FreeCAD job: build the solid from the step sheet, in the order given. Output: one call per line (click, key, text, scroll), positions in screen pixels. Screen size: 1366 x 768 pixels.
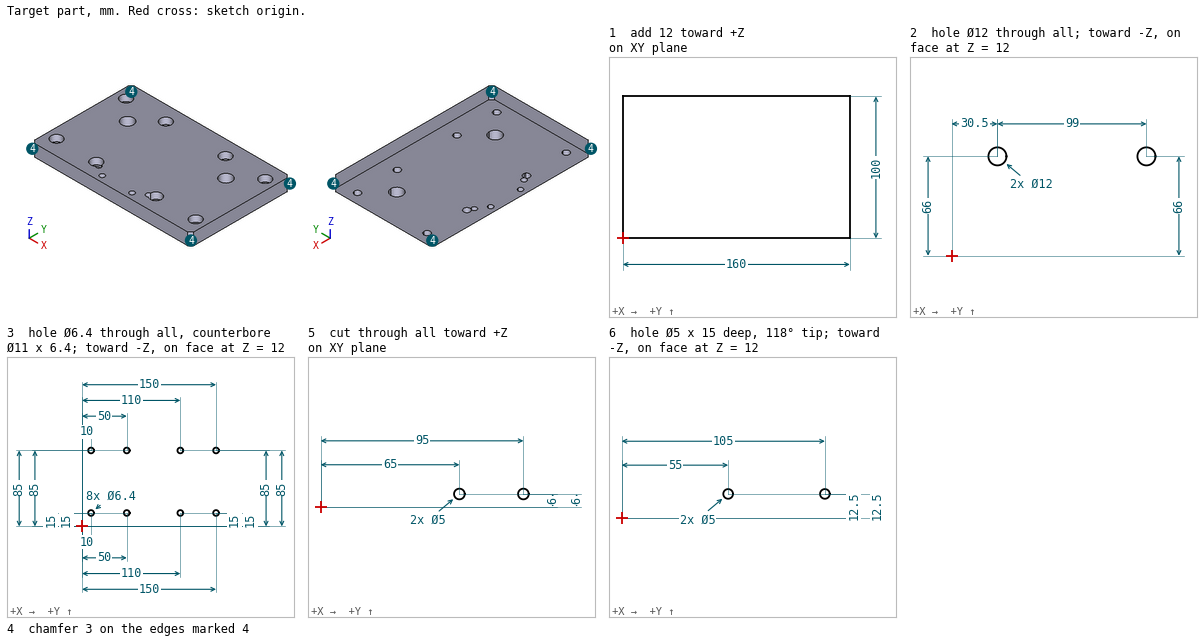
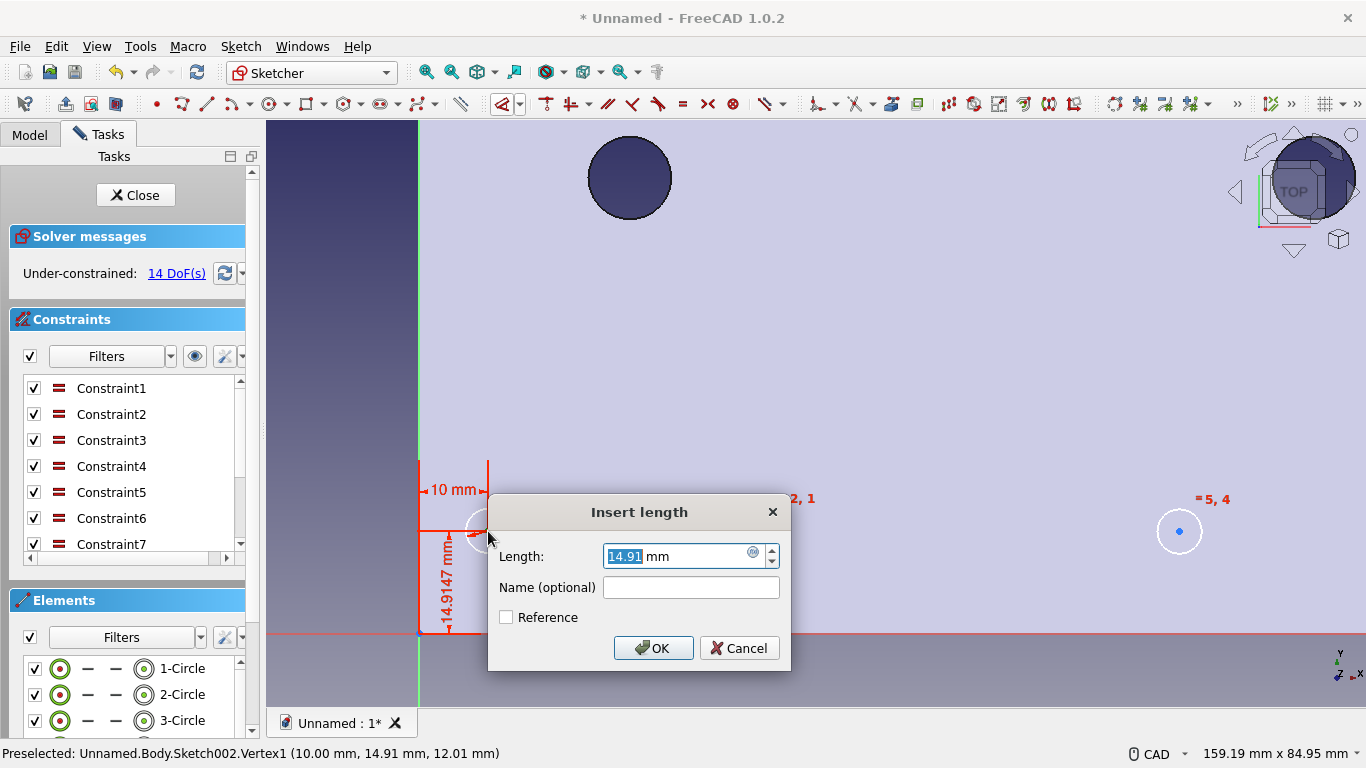
text(15)
key(Return)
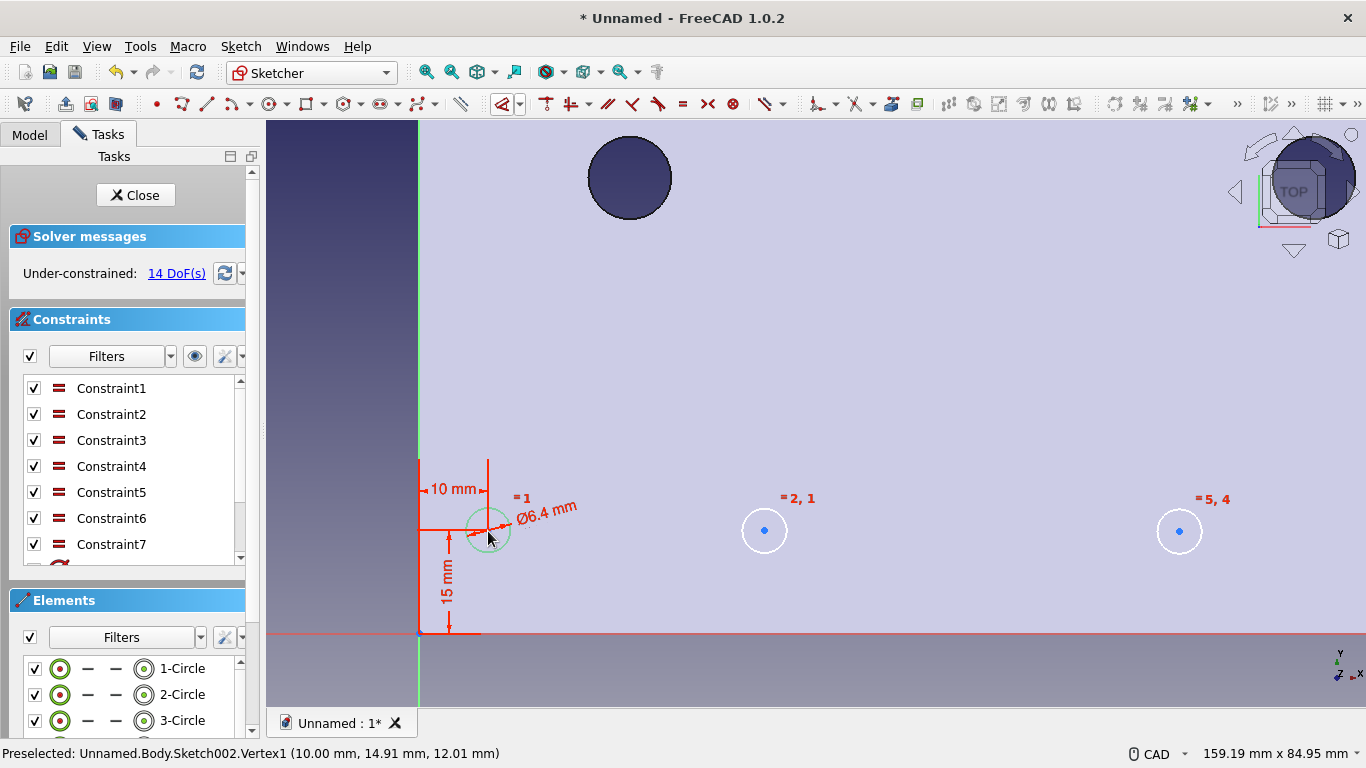
click(765, 531)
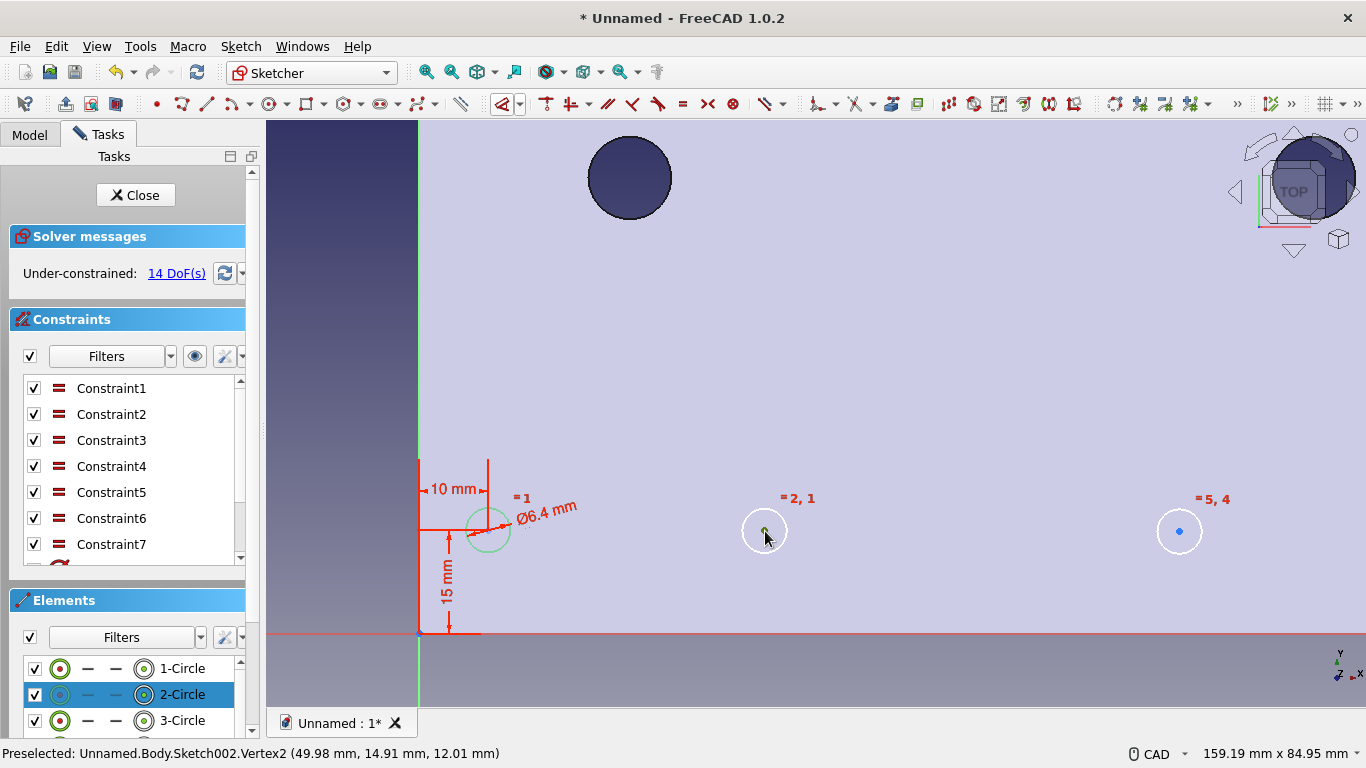
key(l)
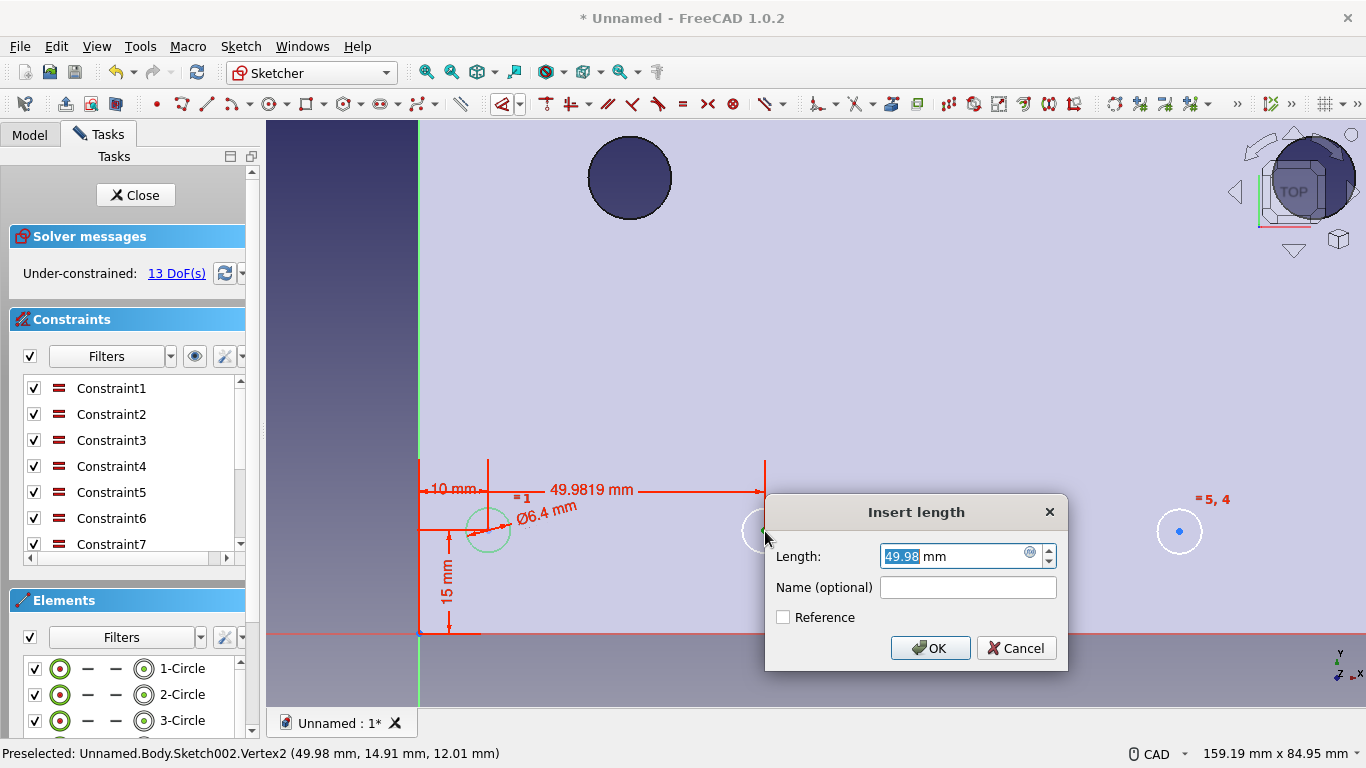
text(50)
key(Return)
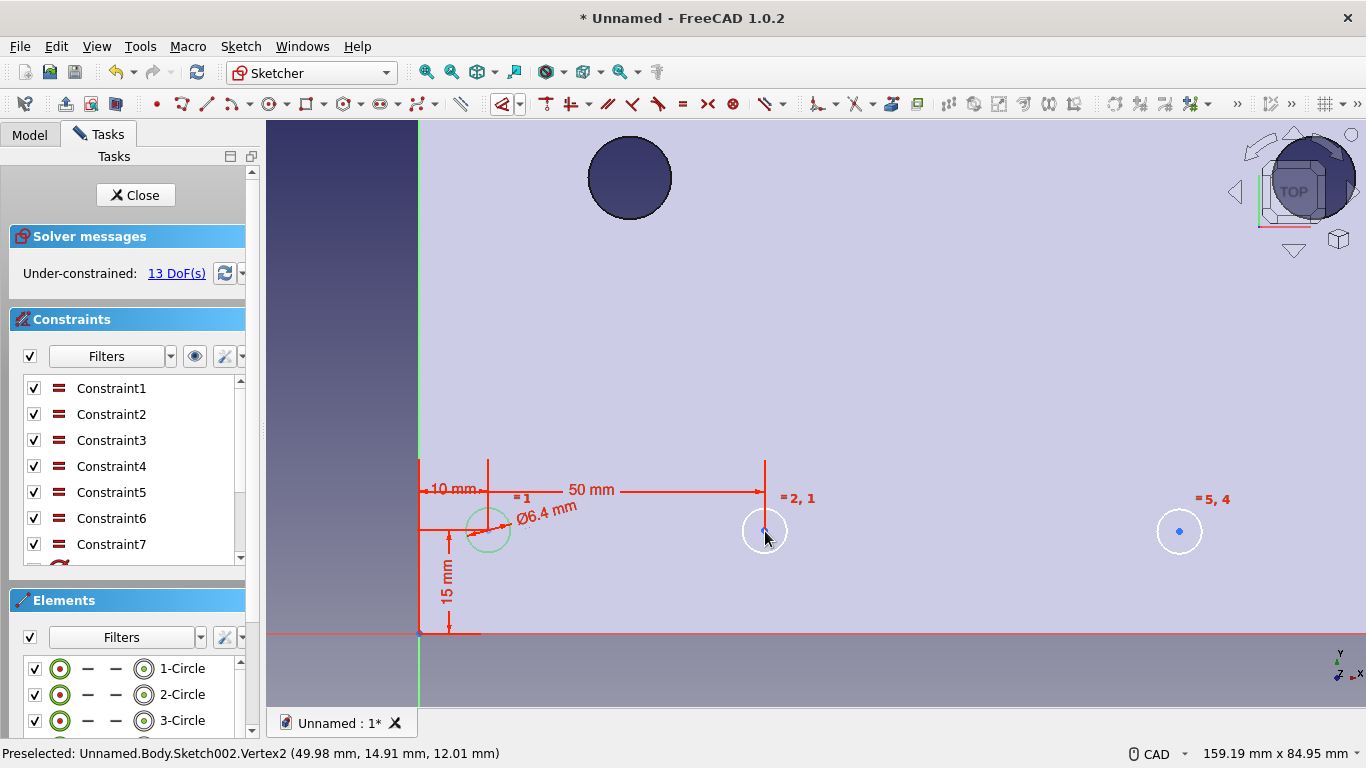
click(765, 531)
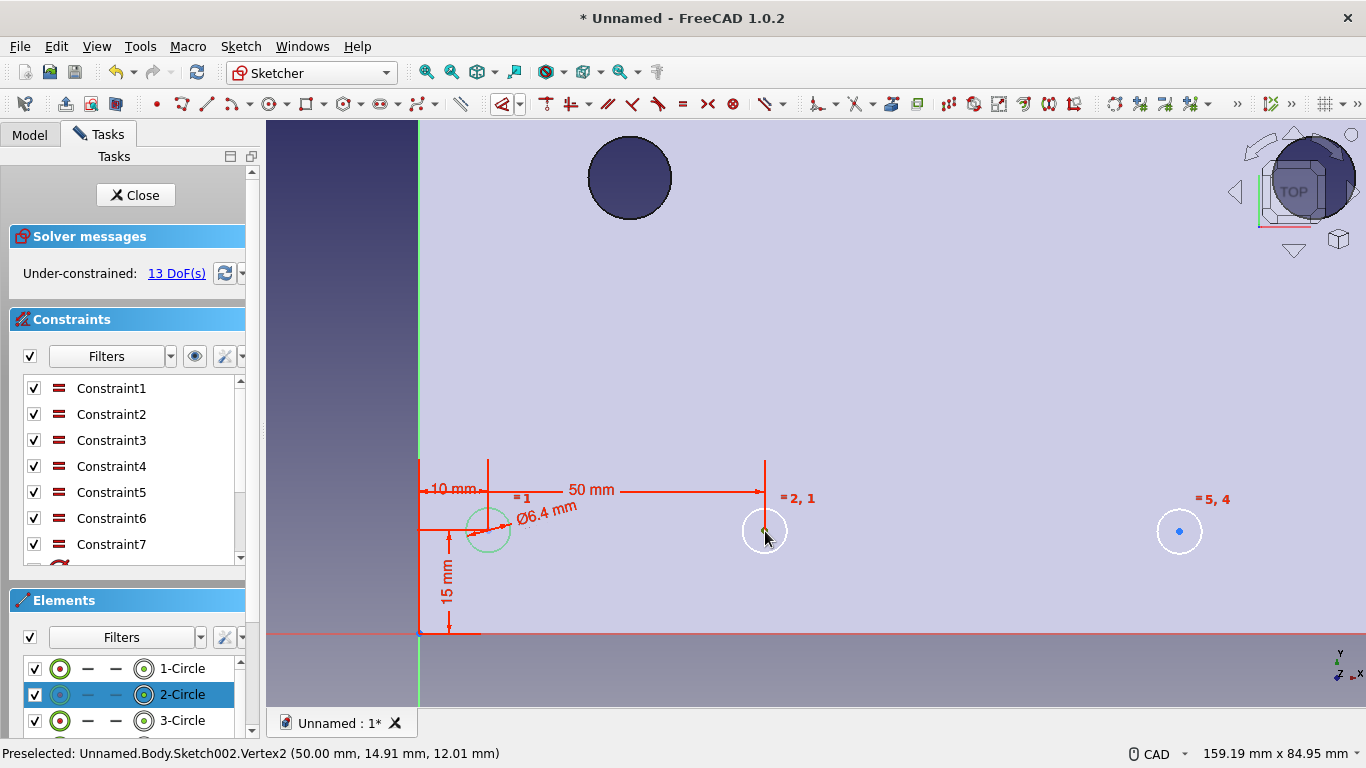
key(i)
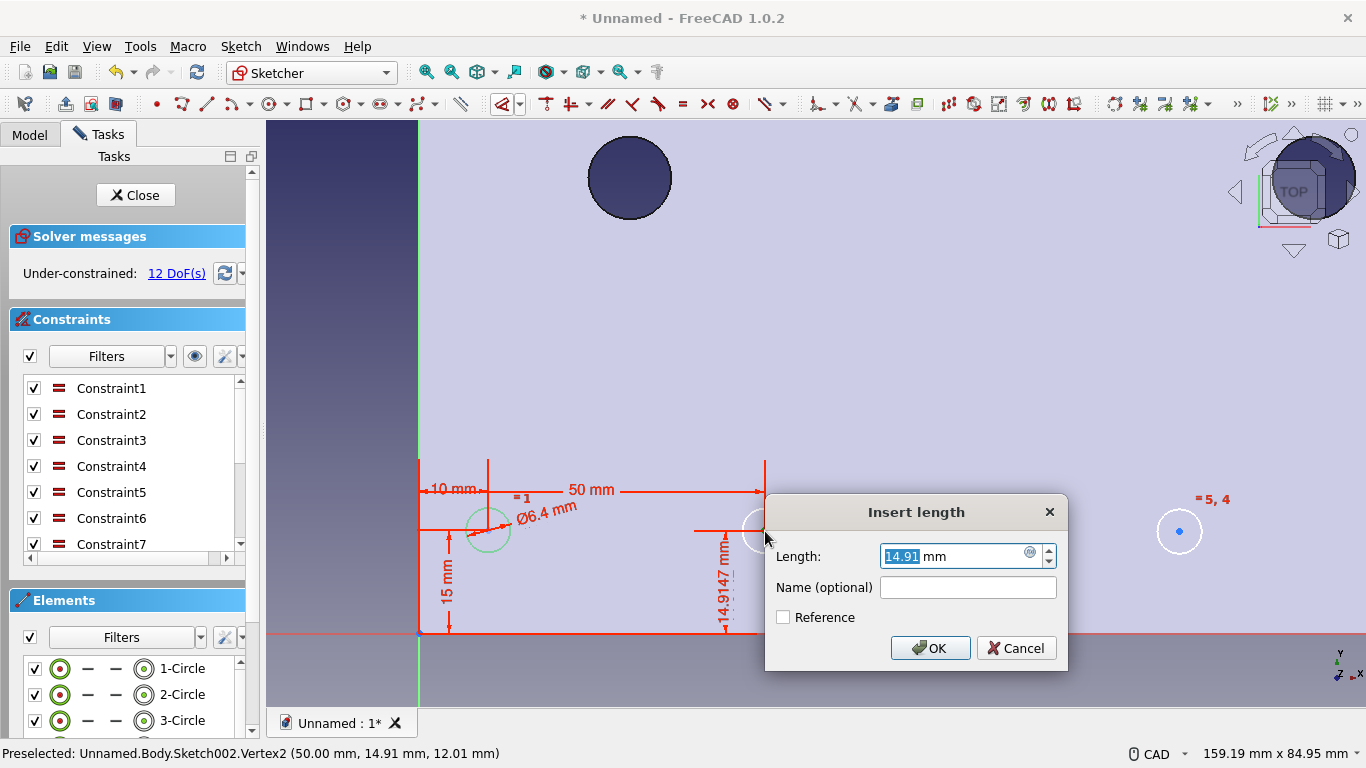
text(15)
key(Return)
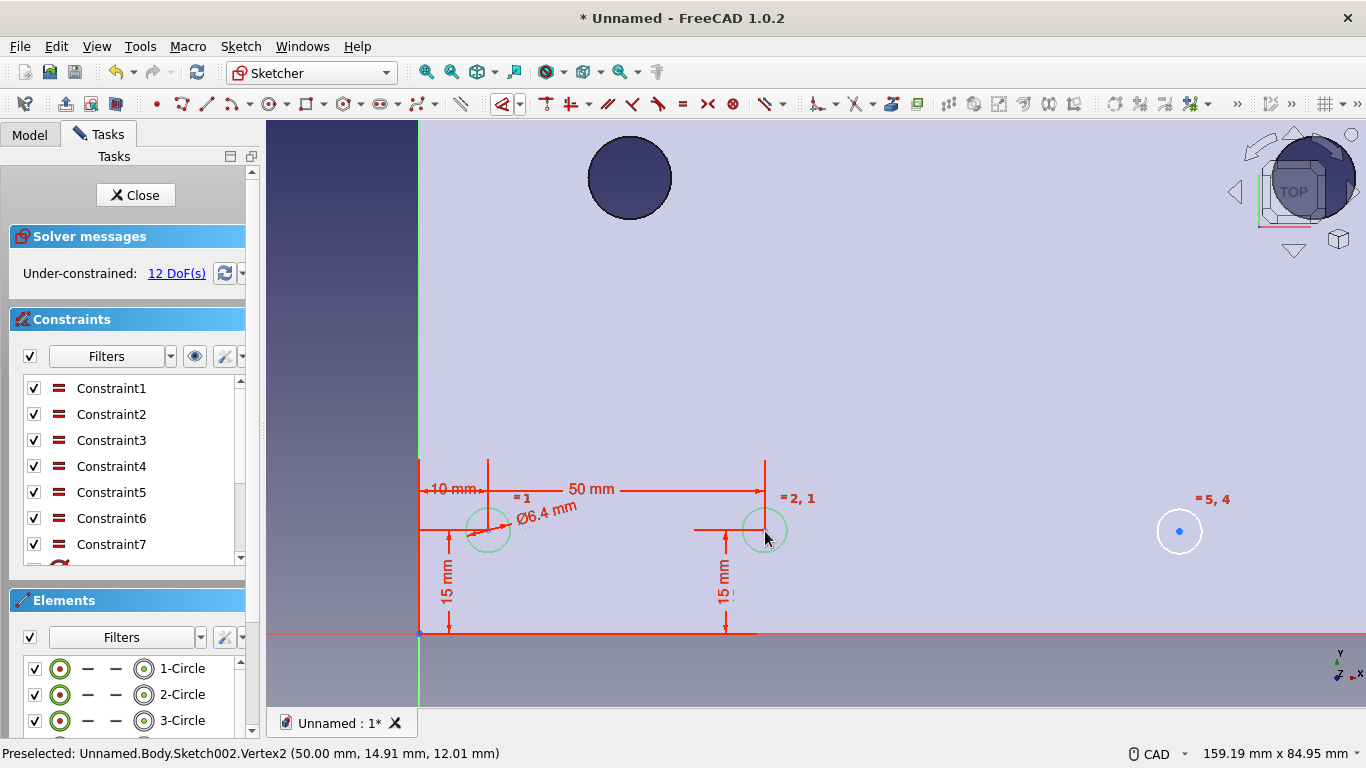
scroll(503, 516, down, 3)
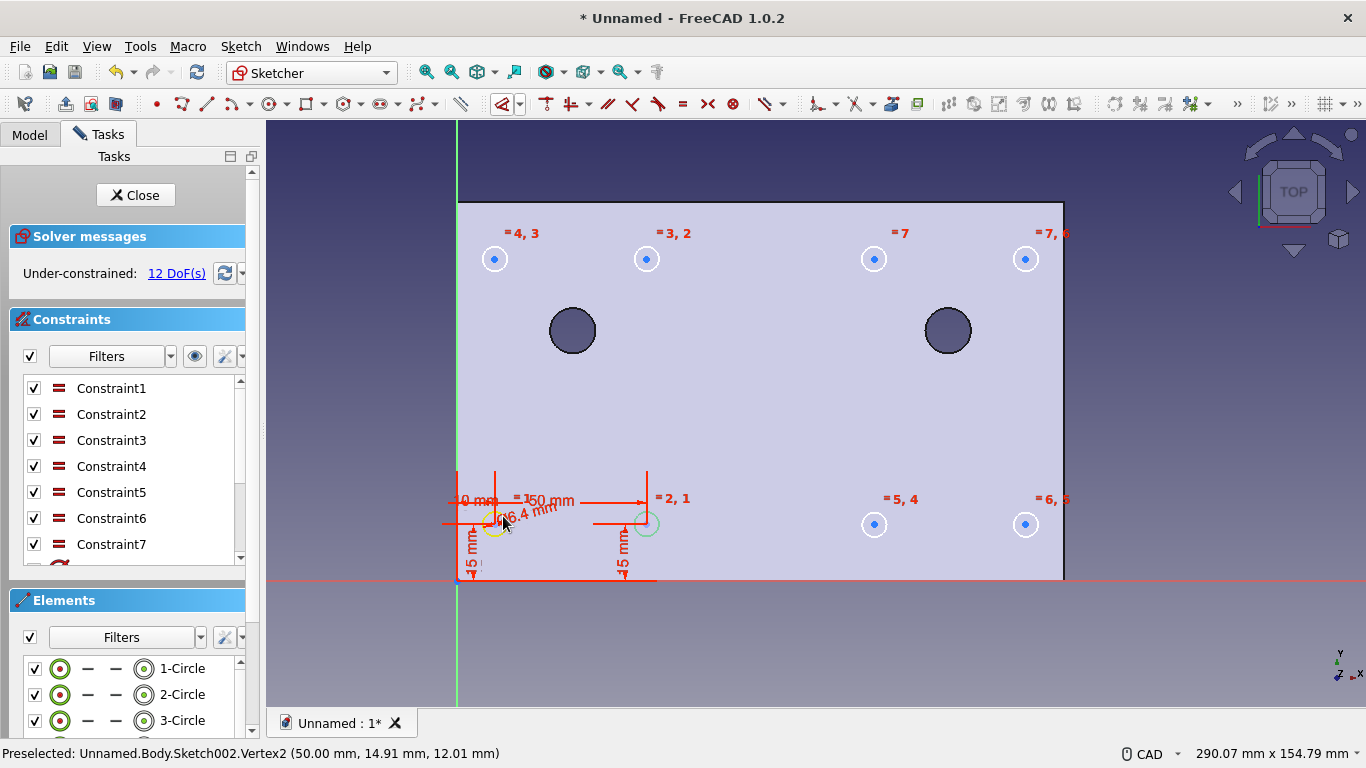
click(647, 259)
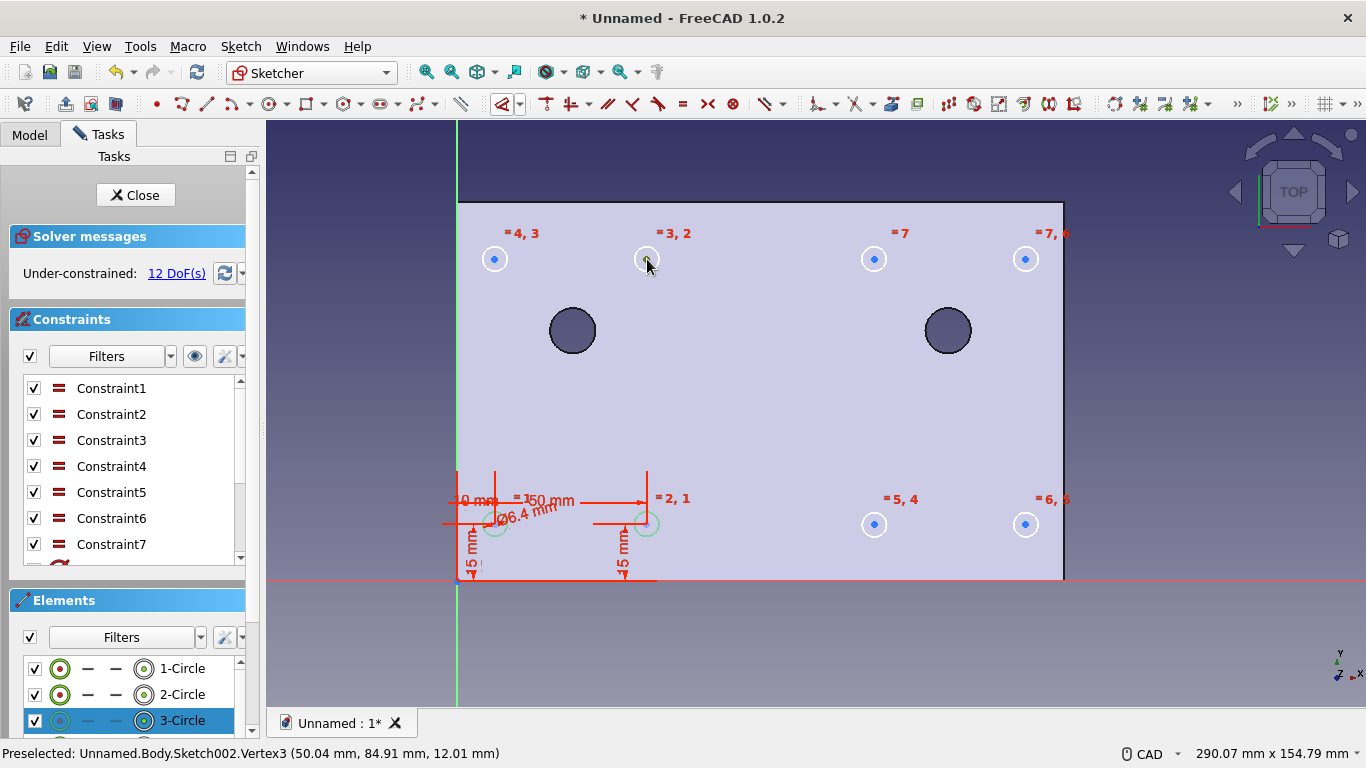
key(l)